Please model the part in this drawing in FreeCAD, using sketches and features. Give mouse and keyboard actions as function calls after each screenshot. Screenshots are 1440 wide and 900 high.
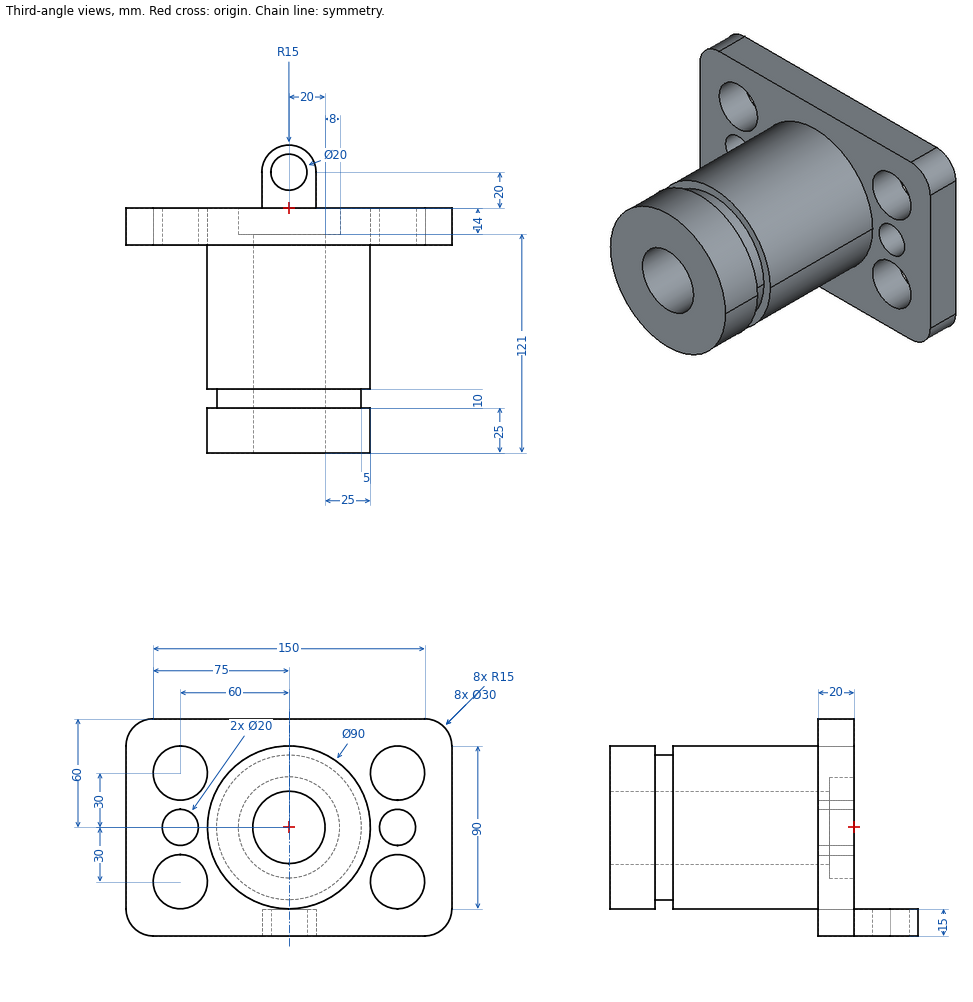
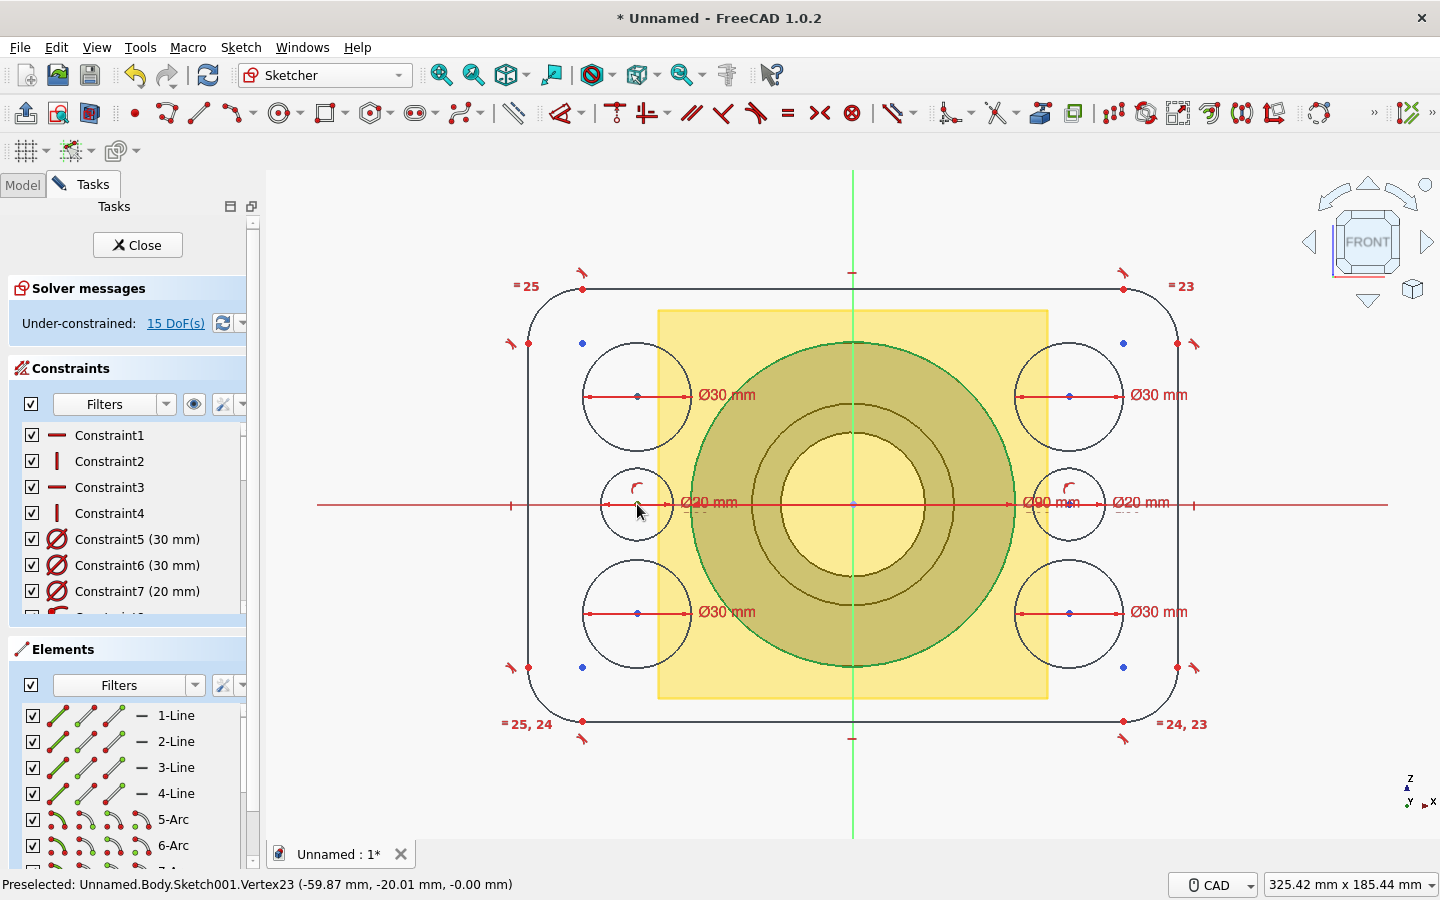
click(670, 114)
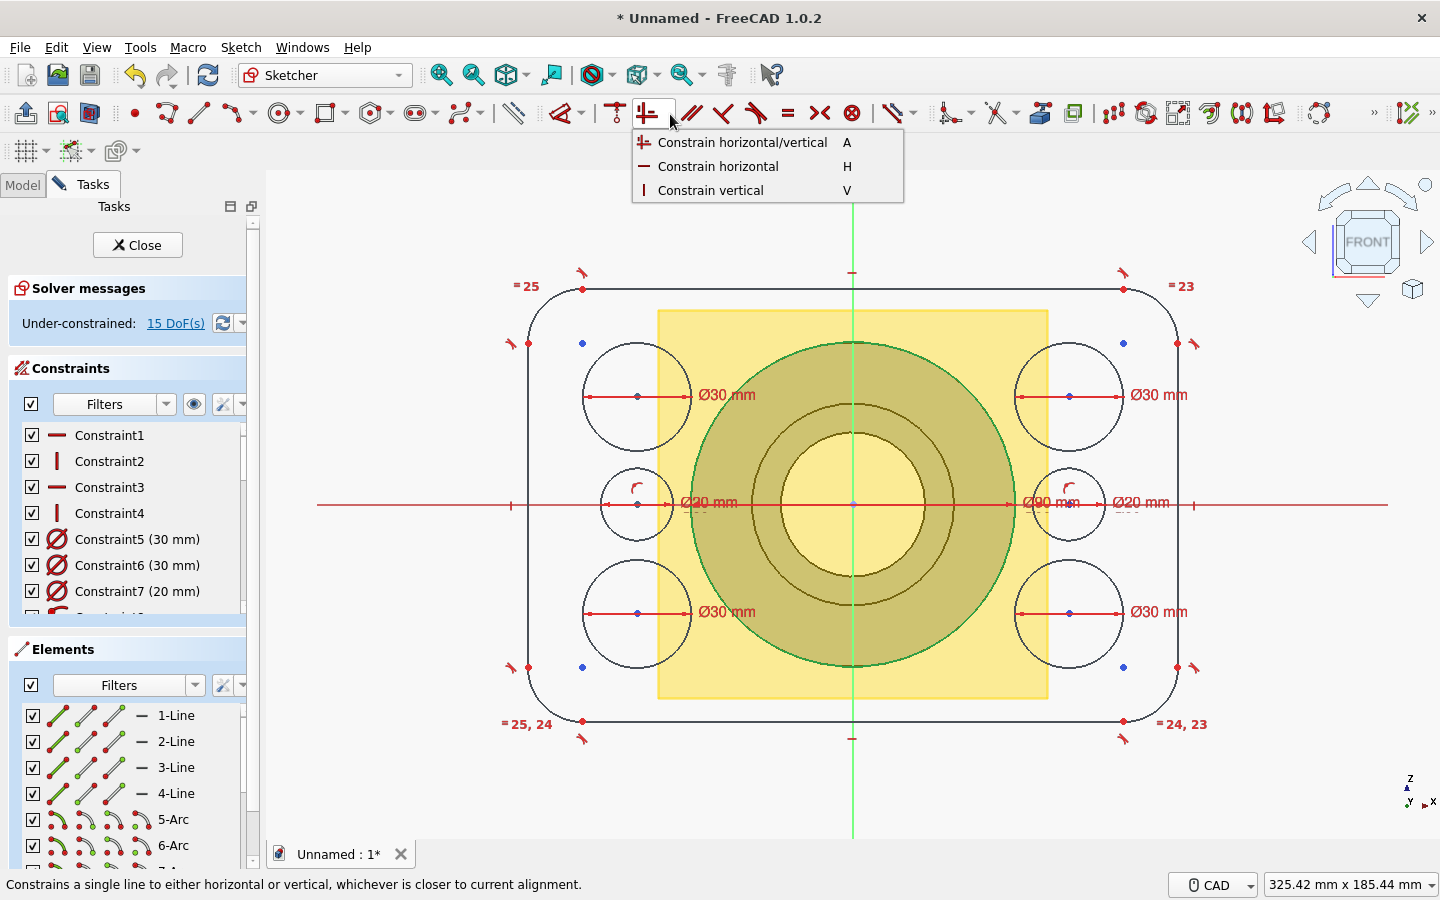
click(768, 190)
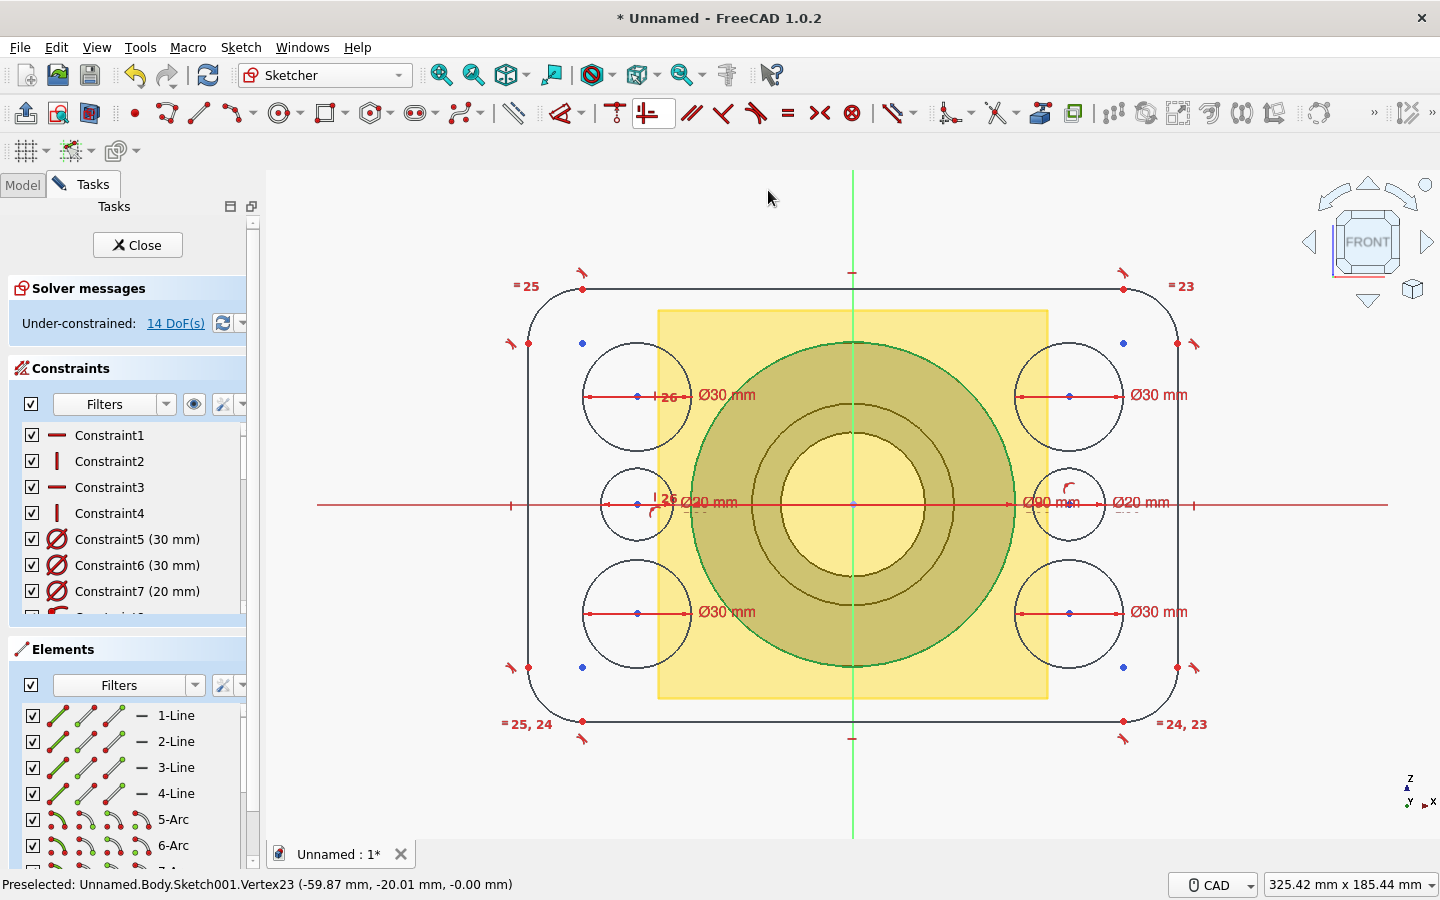
click(637, 504)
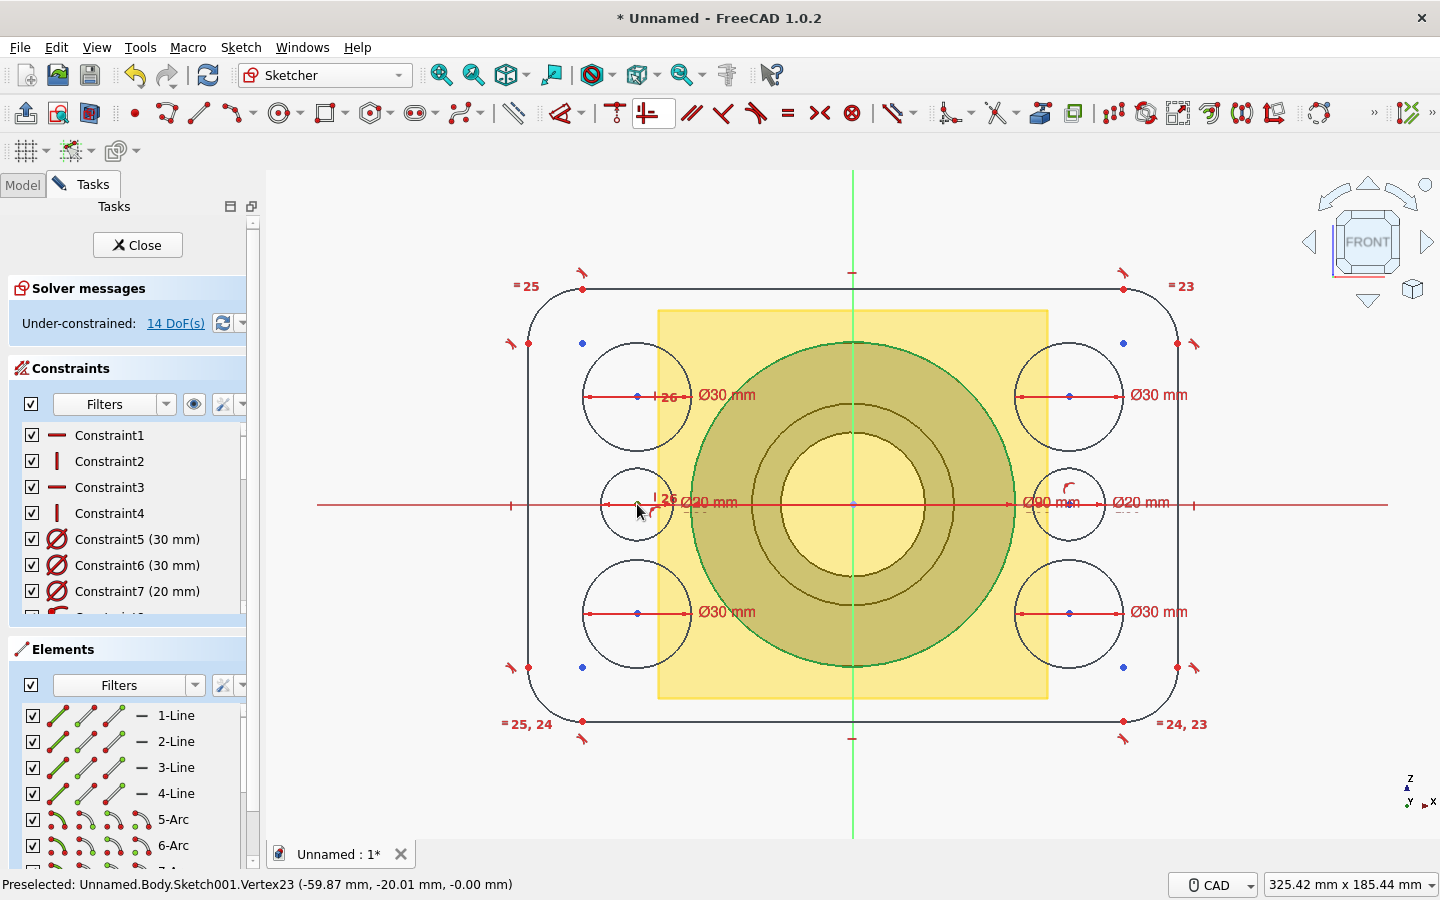
click(637, 614)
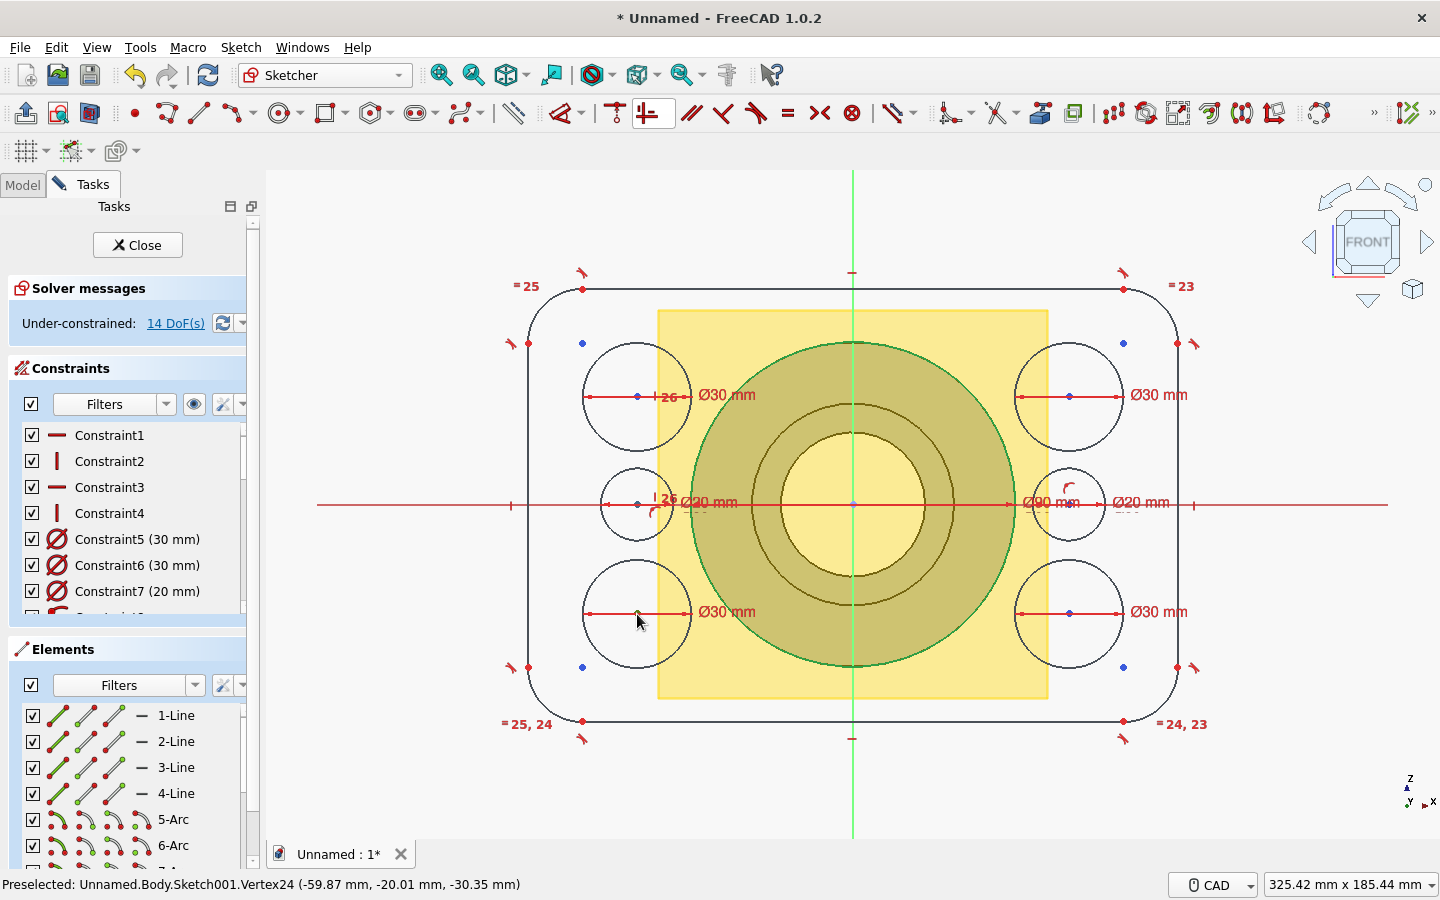
key(v)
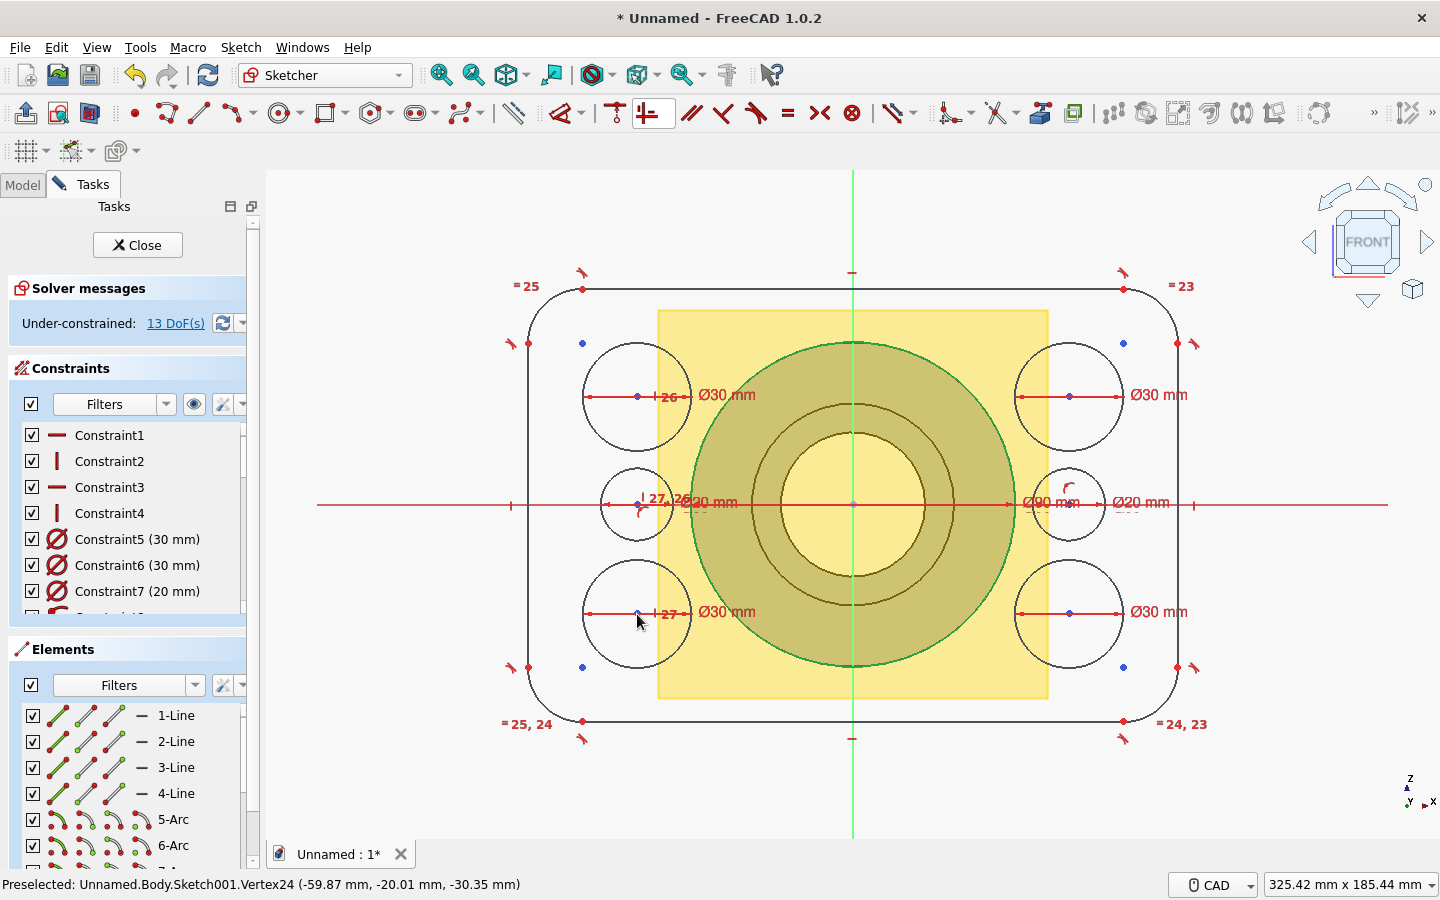
click(1069, 397)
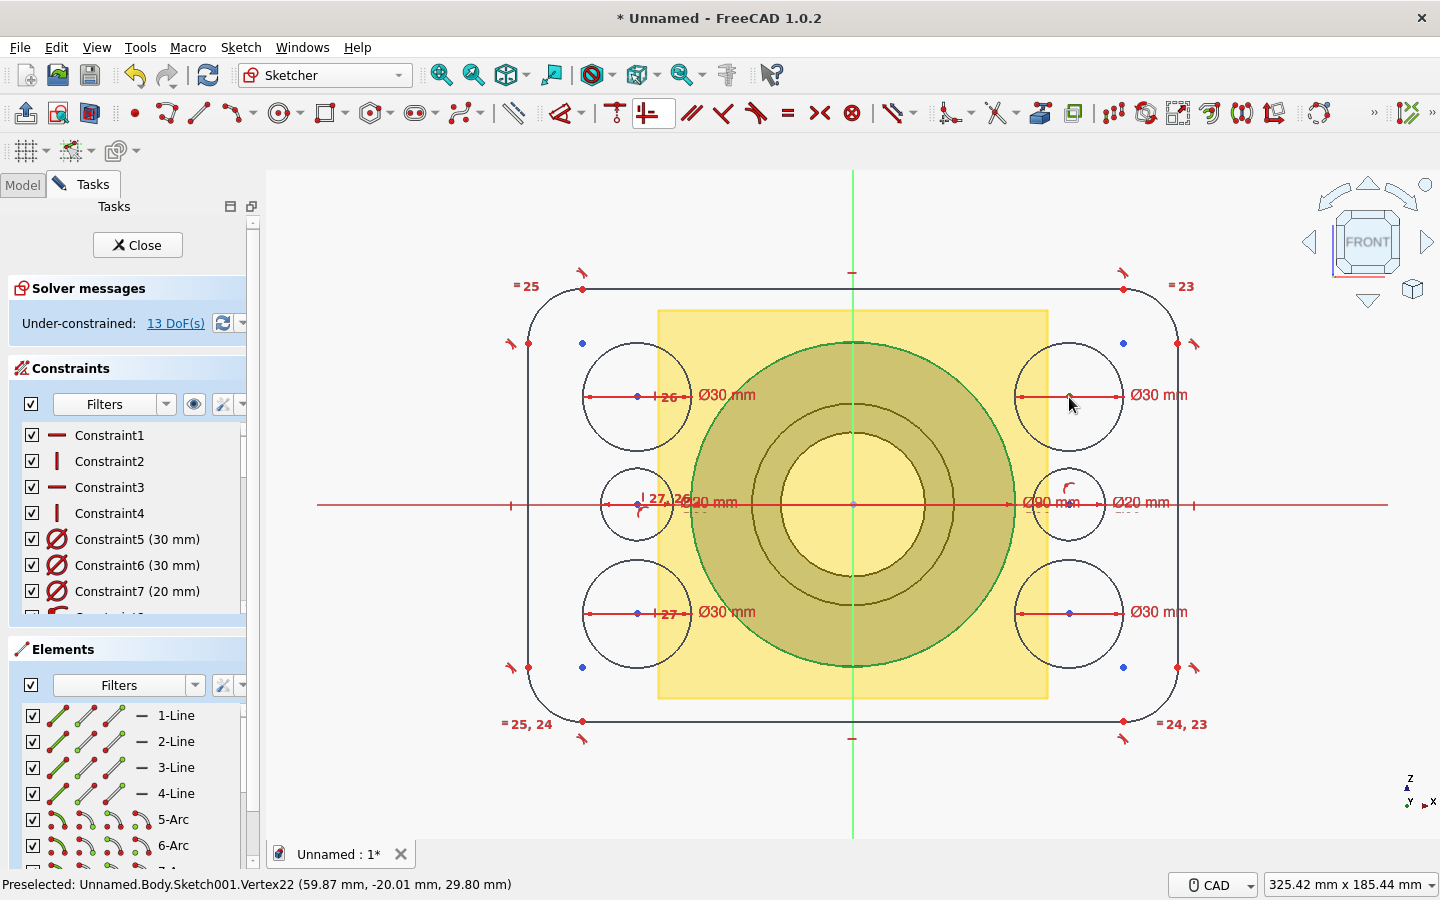
click(1069, 504)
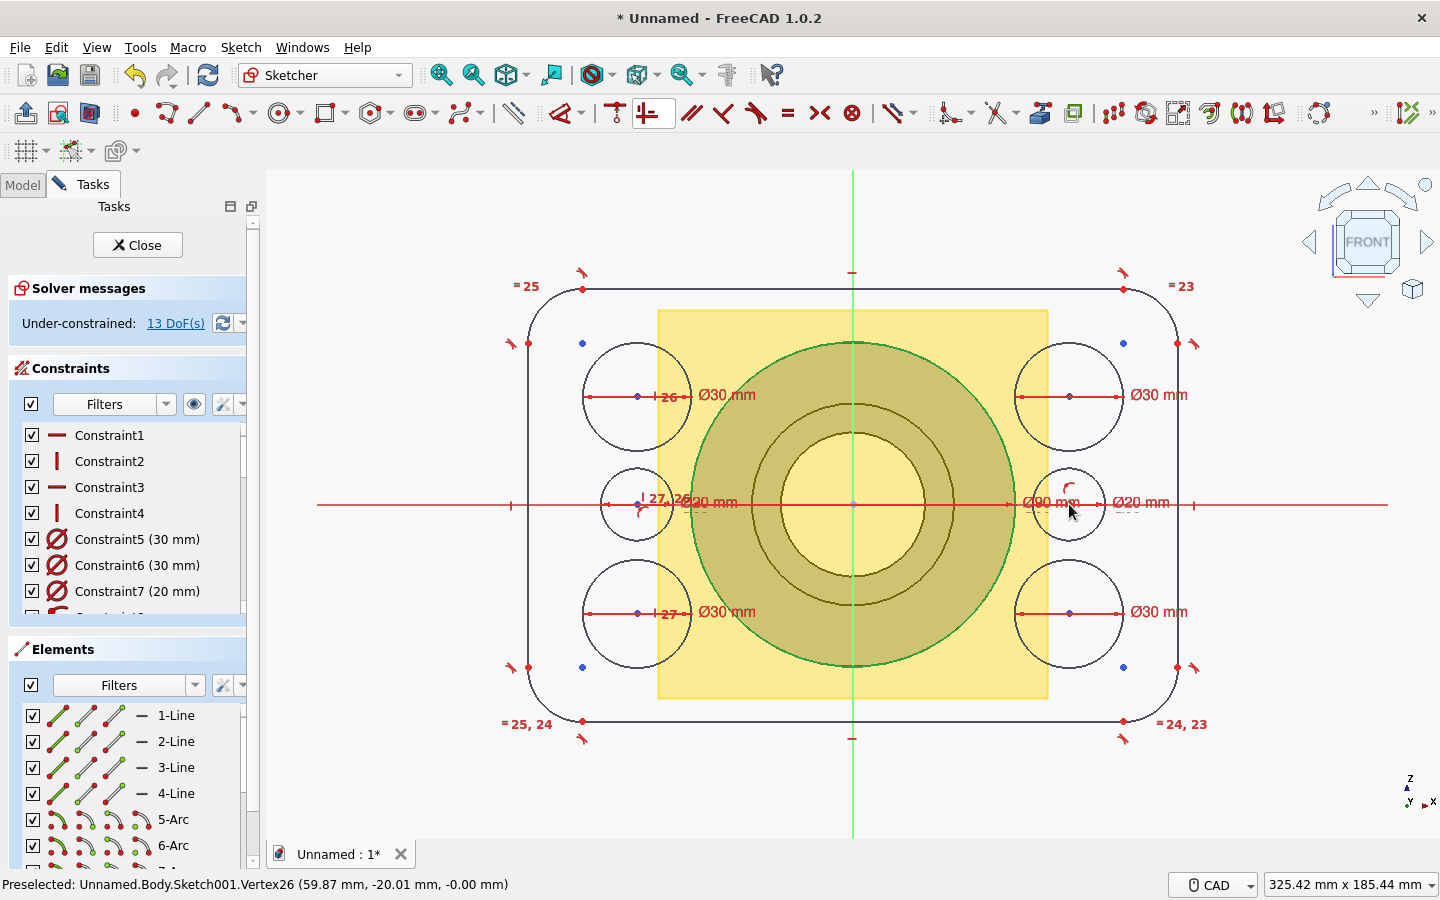
key(v)